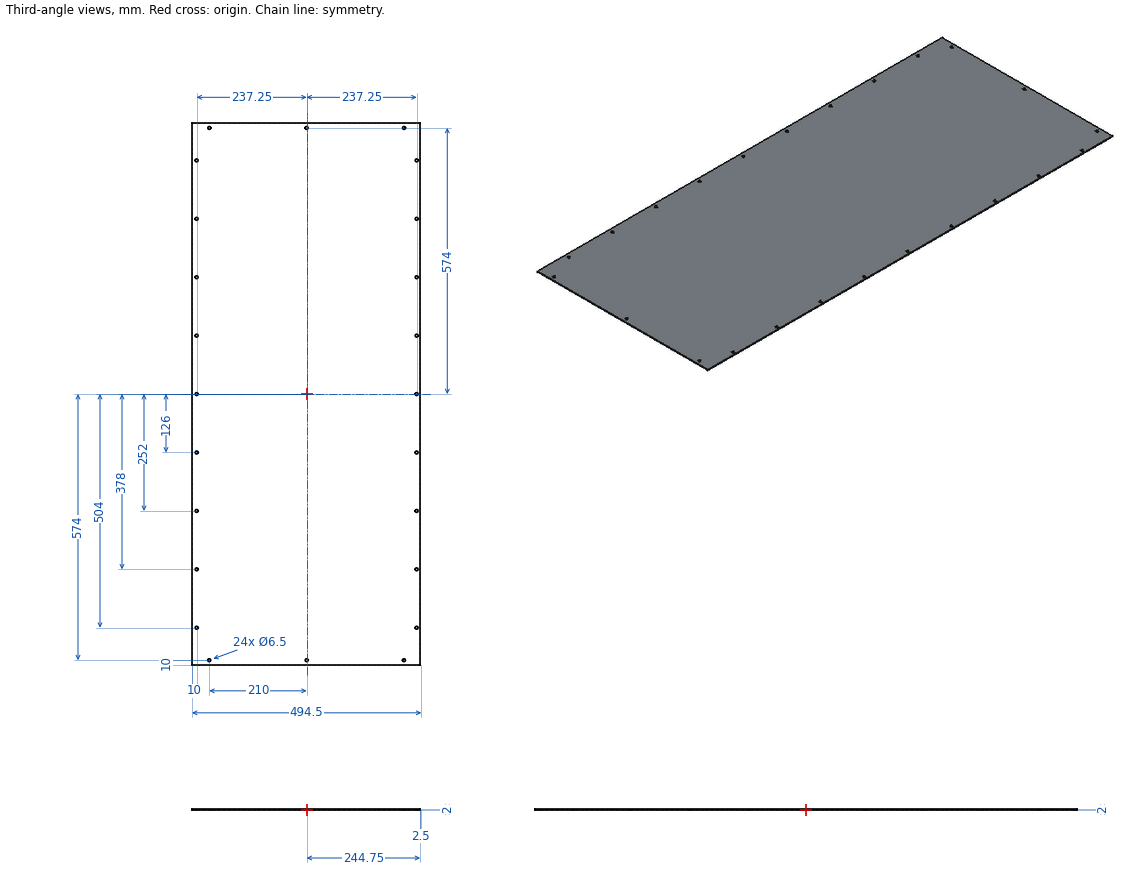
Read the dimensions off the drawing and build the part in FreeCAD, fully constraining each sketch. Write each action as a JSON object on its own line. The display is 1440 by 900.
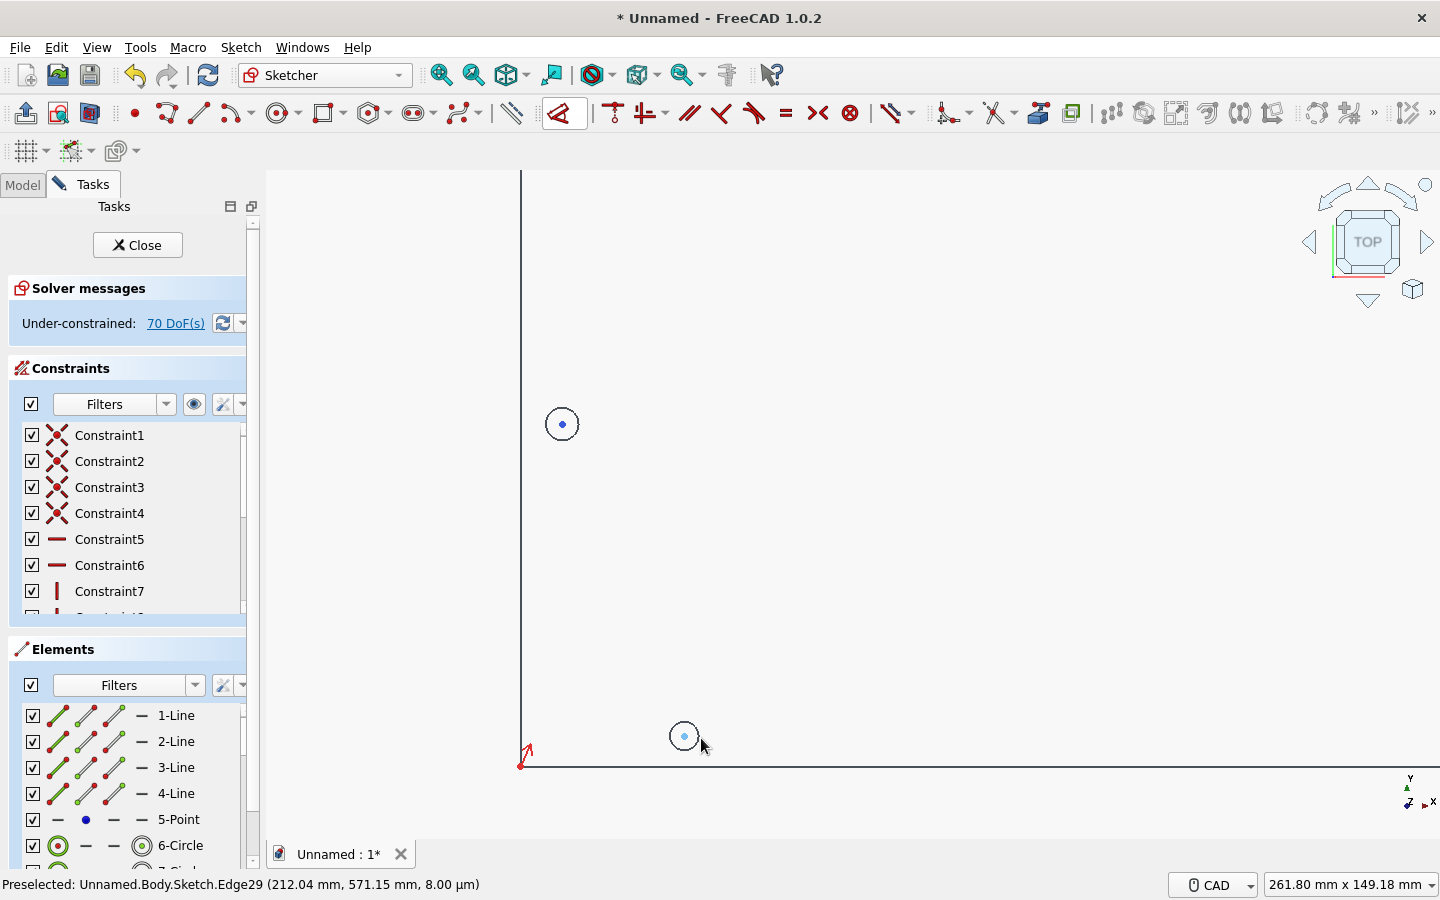
{"action": "left_click", "coordinate": [694, 726]}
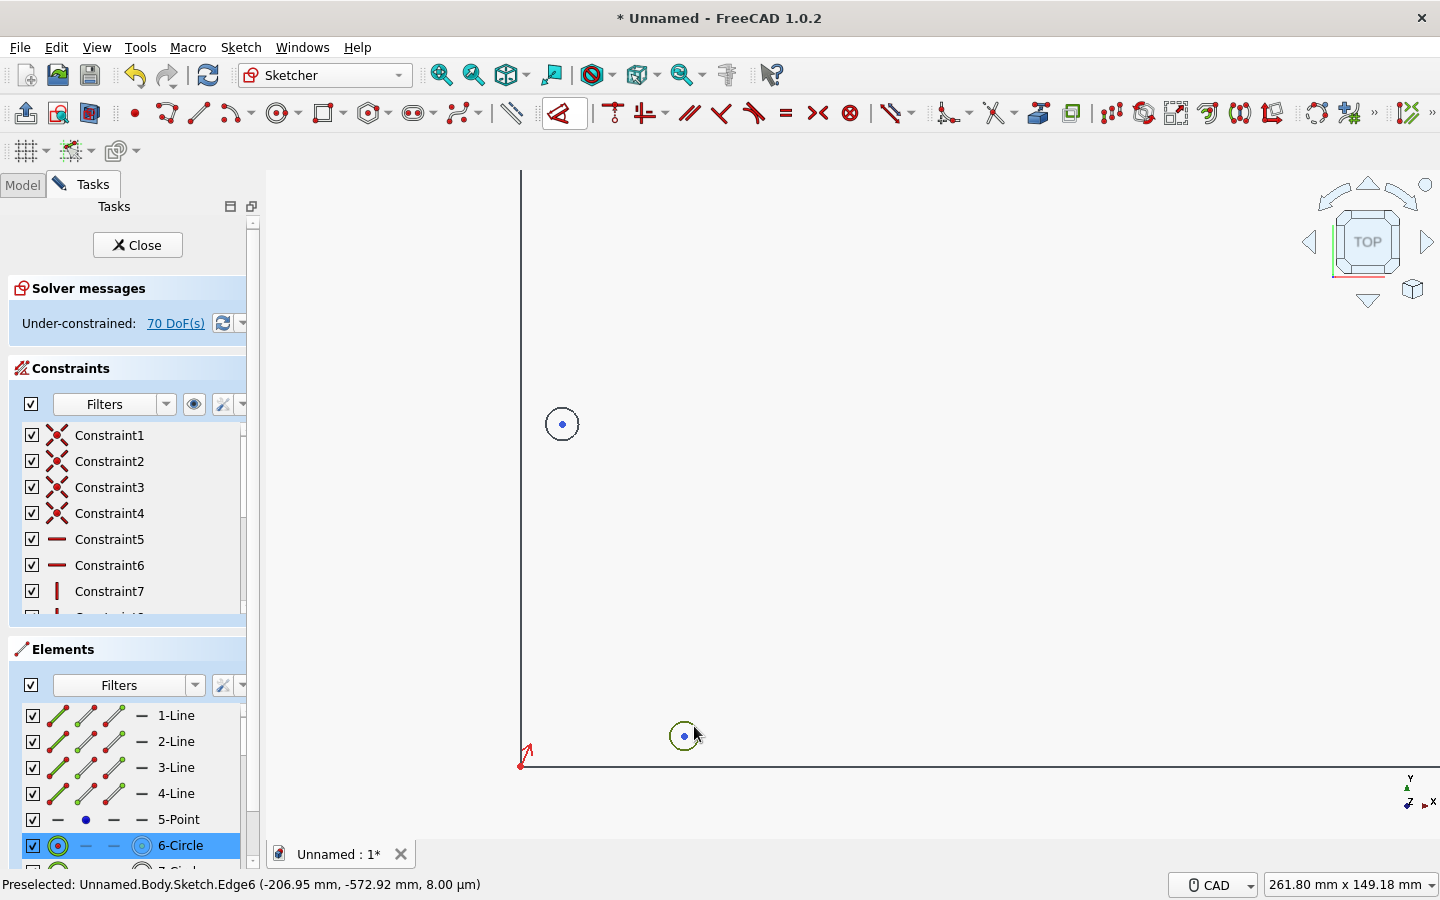
{"action": "left_click", "coordinate": [574, 413]}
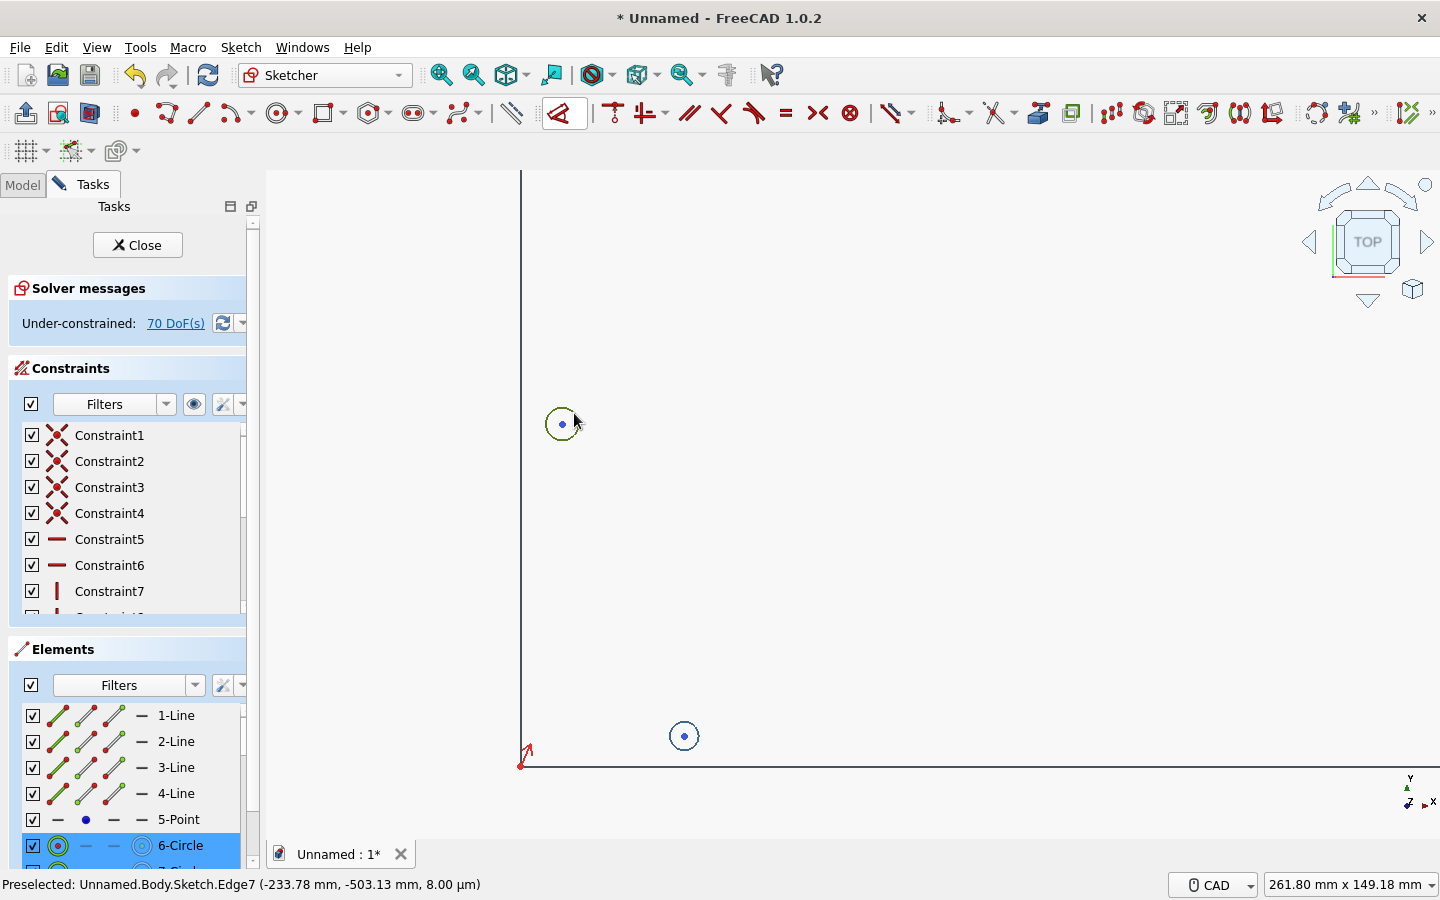
{"action": "scroll", "coordinate": [701, 738], "scroll_direction": "down", "scroll_amount": 12}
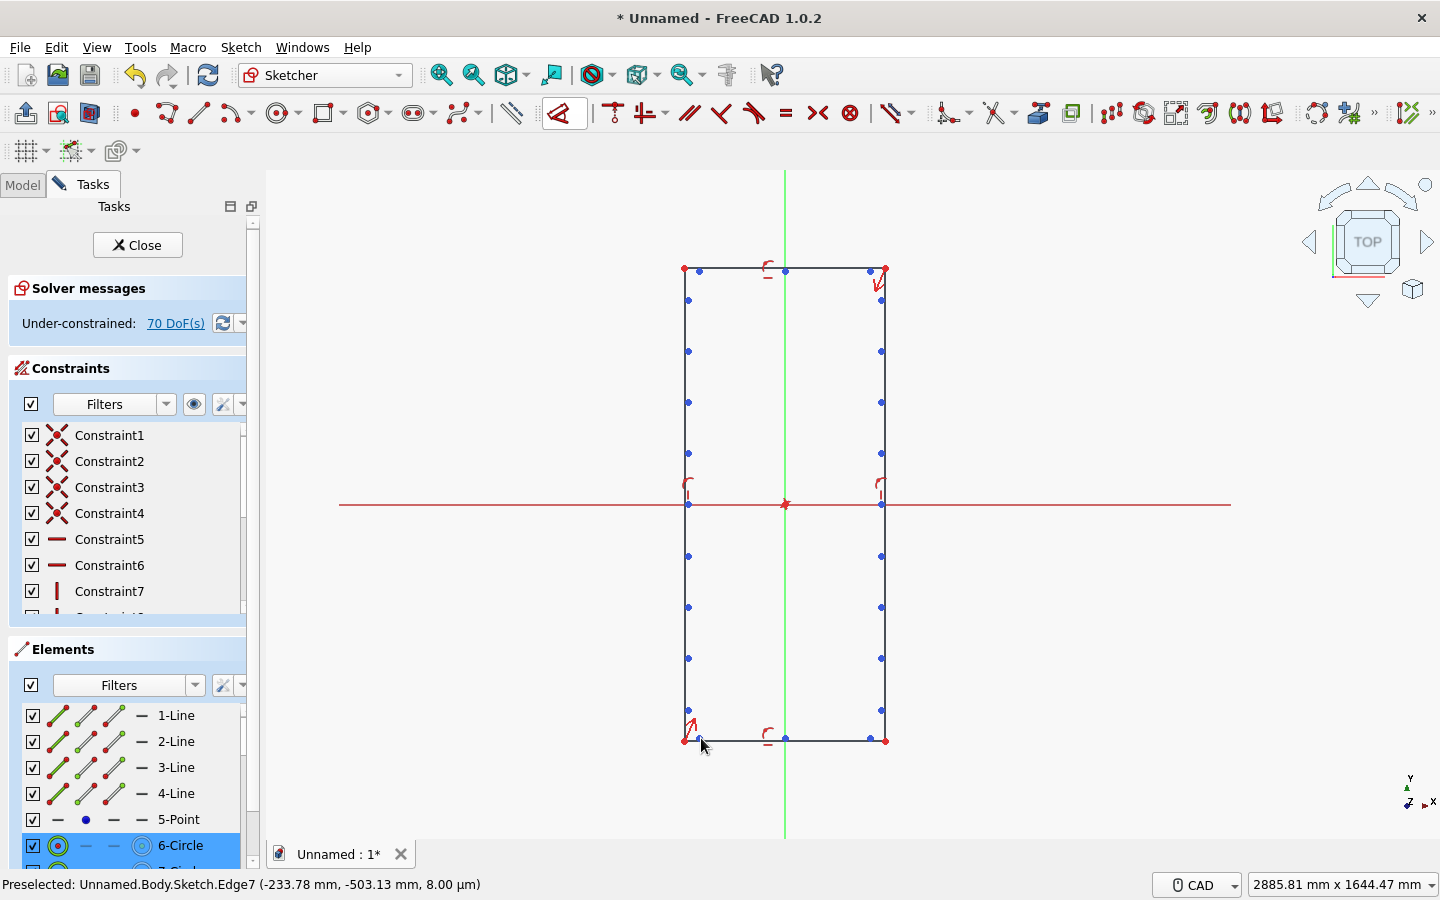
{"action": "scroll", "coordinate": [690, 658], "scroll_direction": "up", "scroll_amount": 12}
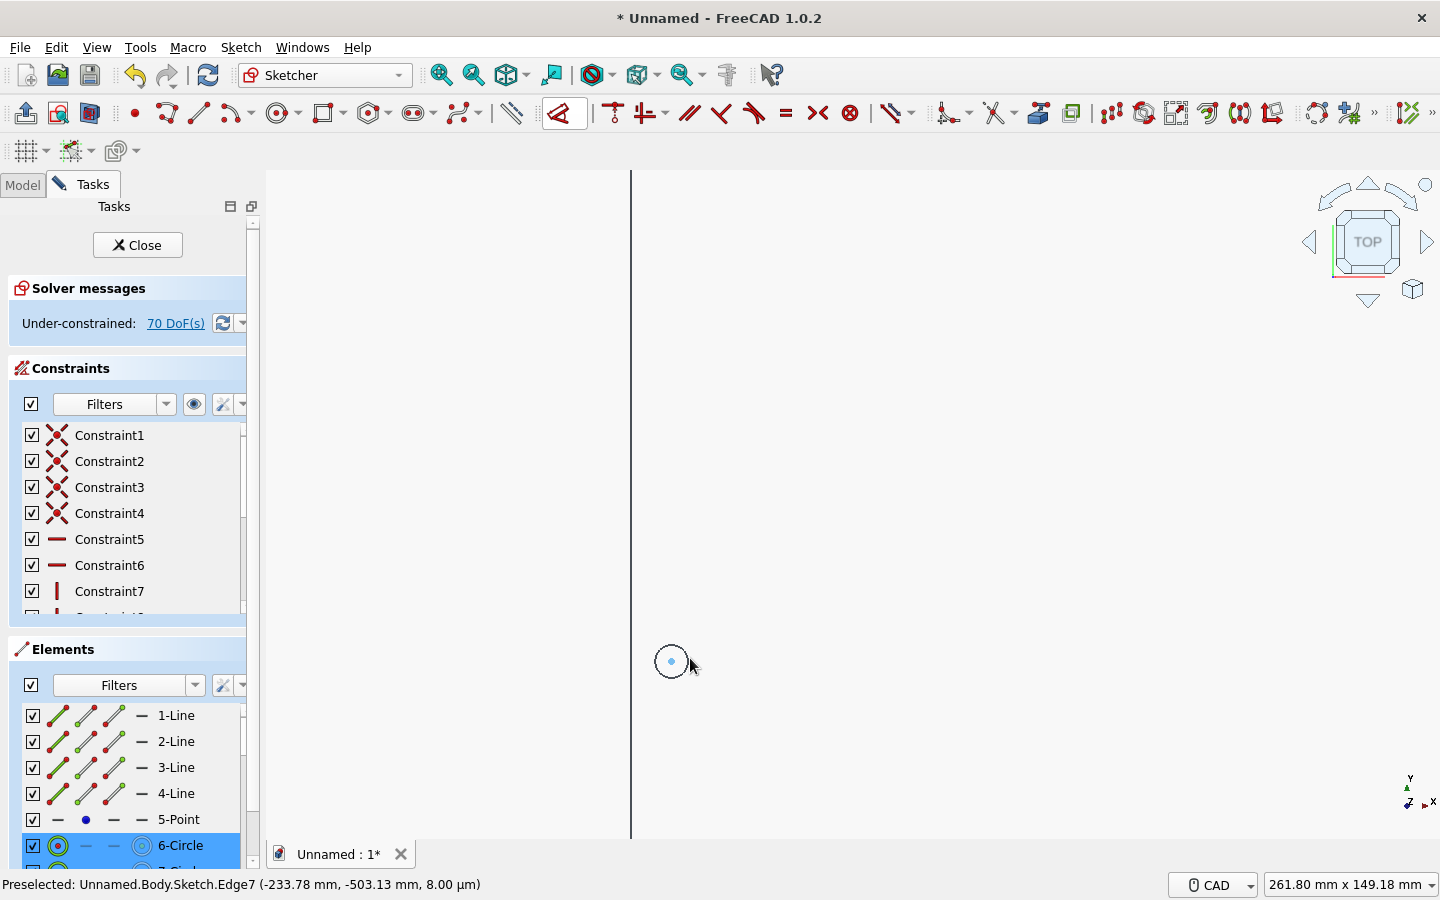
{"action": "left_click", "coordinate": [683, 650]}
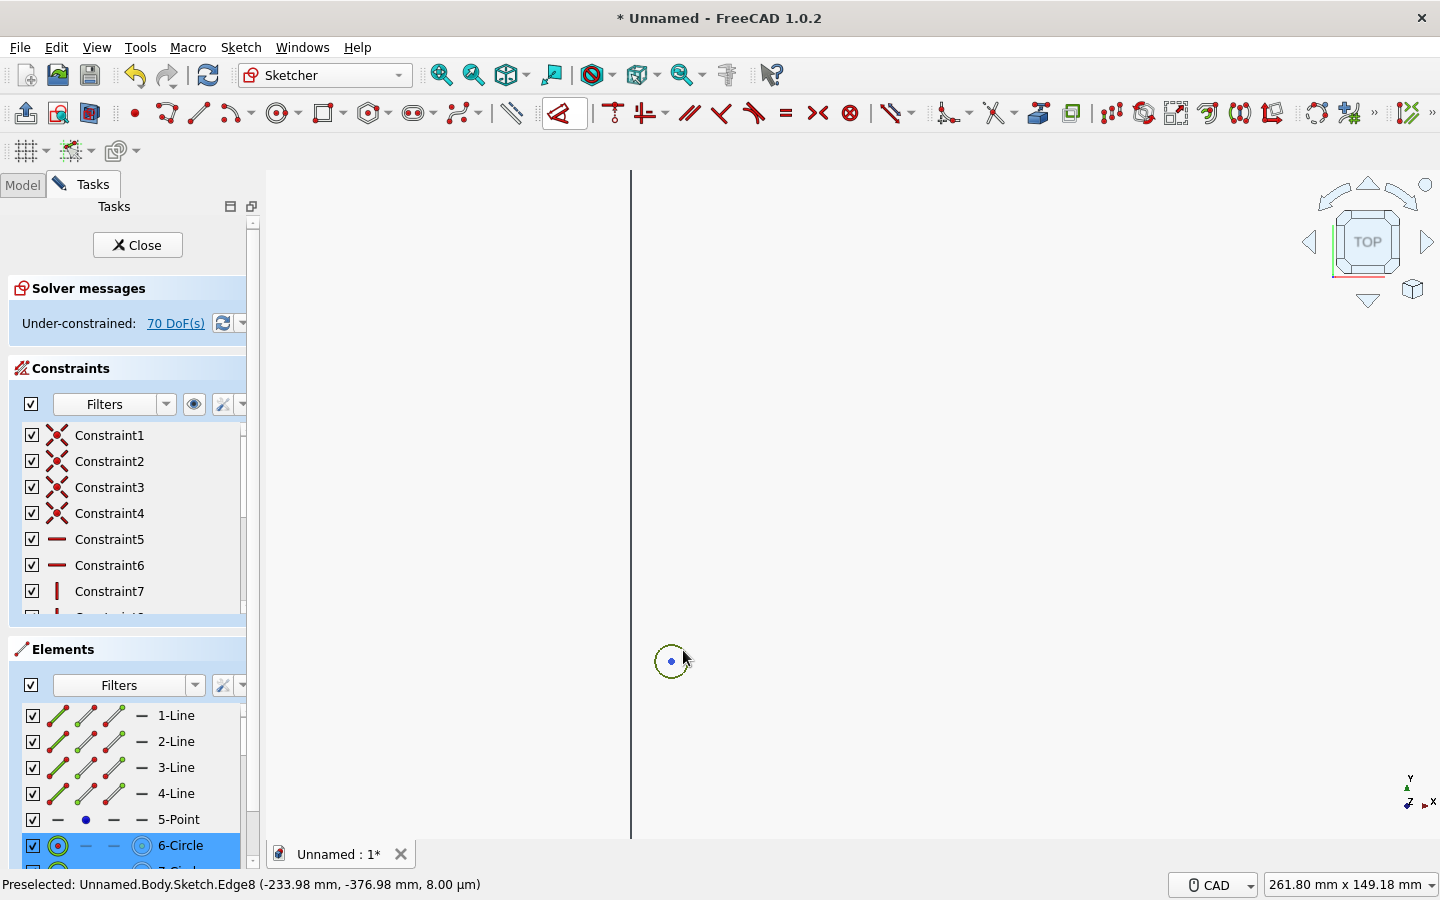
{"action": "scroll", "coordinate": [690, 658], "scroll_direction": "down", "scroll_amount": 12}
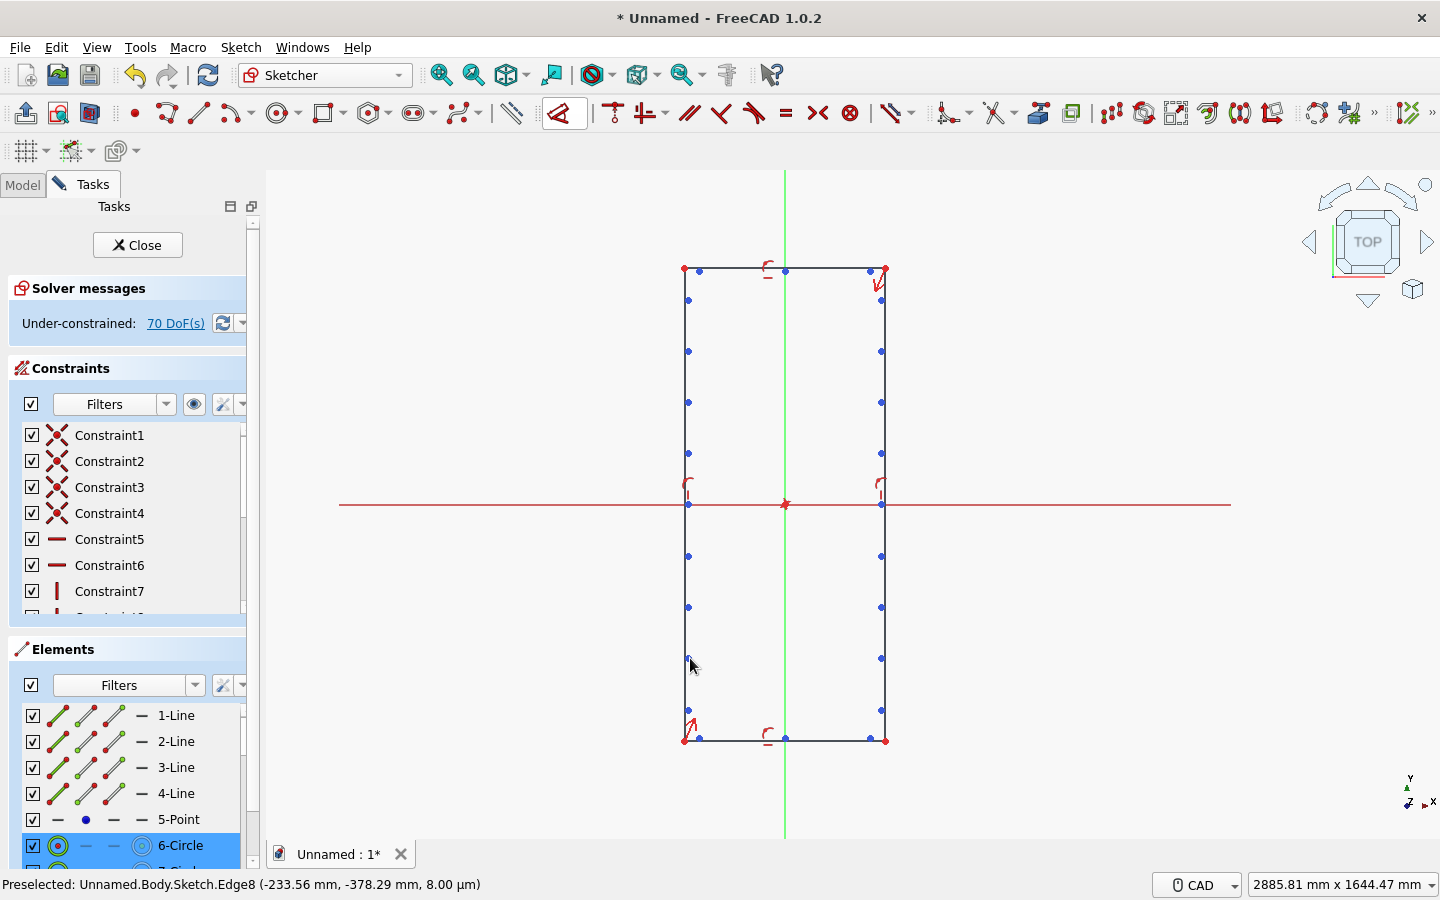
{"action": "scroll", "coordinate": [690, 607], "scroll_direction": "up", "scroll_amount": 12}